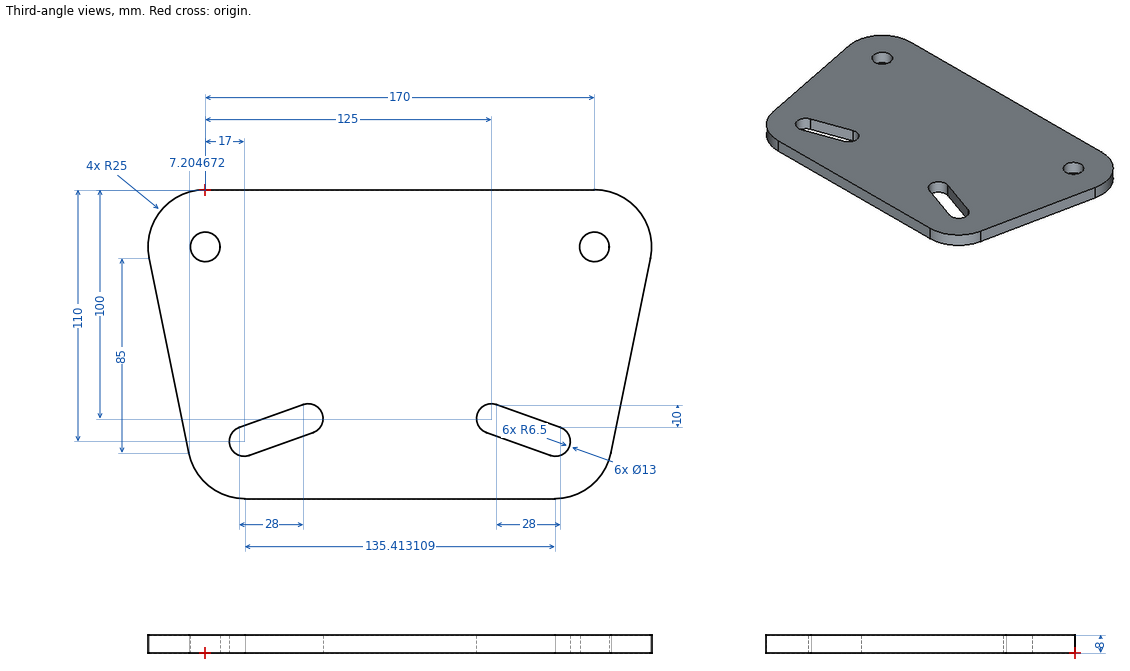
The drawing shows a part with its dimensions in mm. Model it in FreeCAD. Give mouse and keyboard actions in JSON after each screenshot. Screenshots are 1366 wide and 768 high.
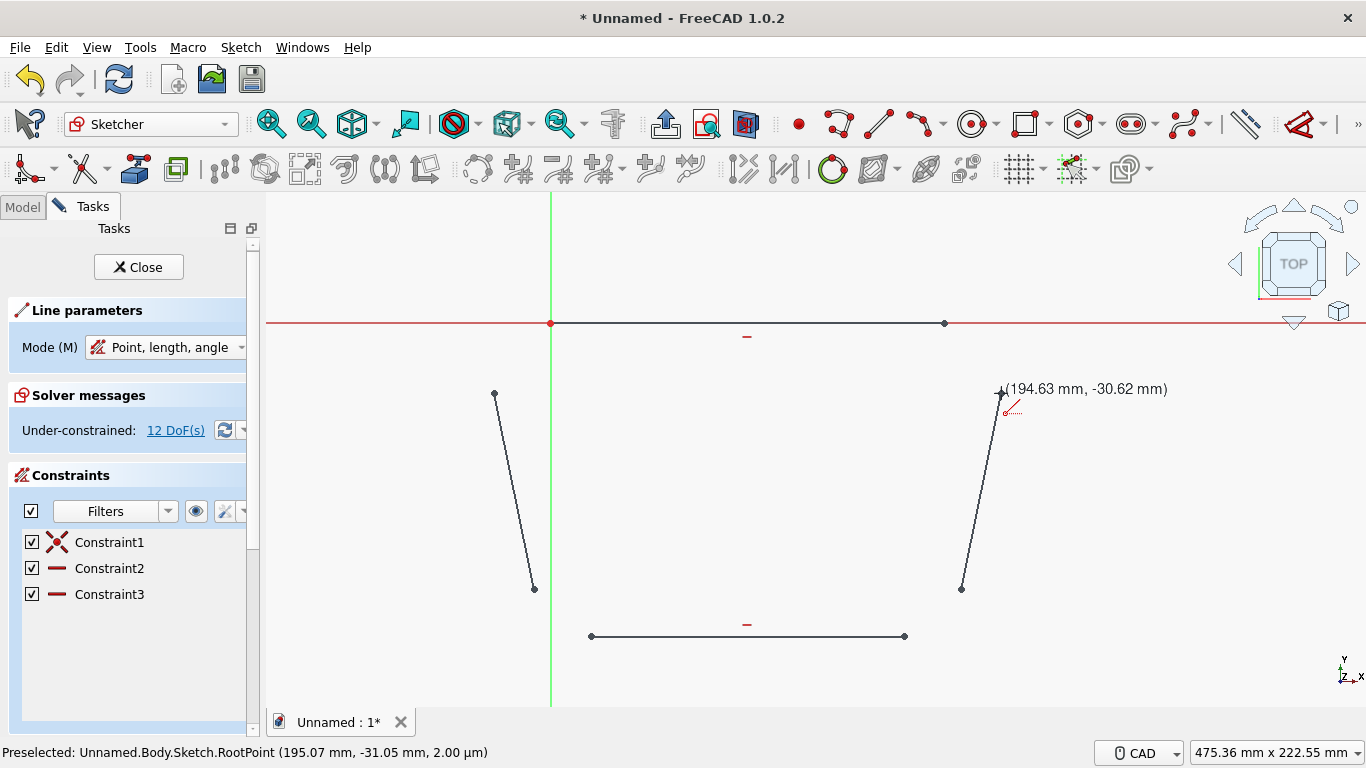
{"action": "left_click", "coordinate": [920, 124]}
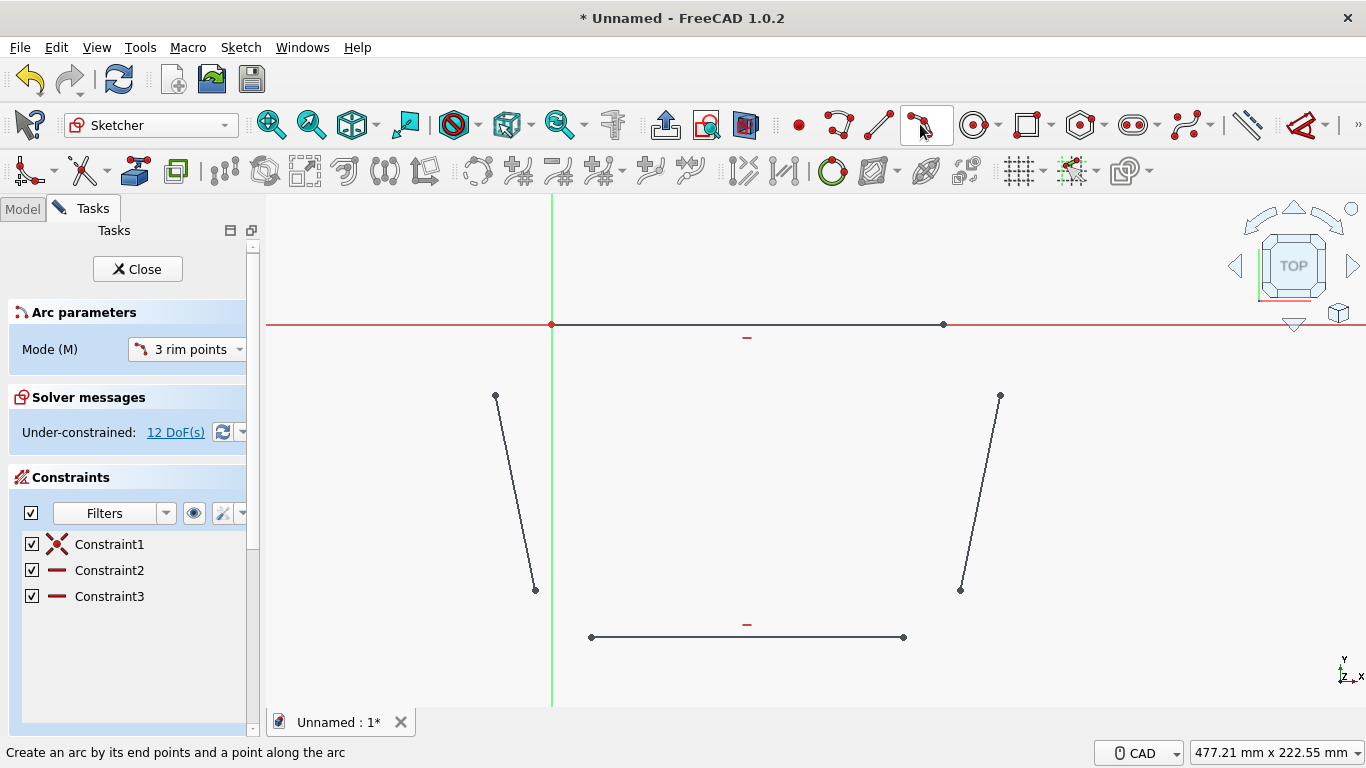
{"action": "left_click", "coordinate": [552, 325]}
{"action": "left_click", "coordinate": [495, 395]}
{"action": "left_click", "coordinate": [507, 346]}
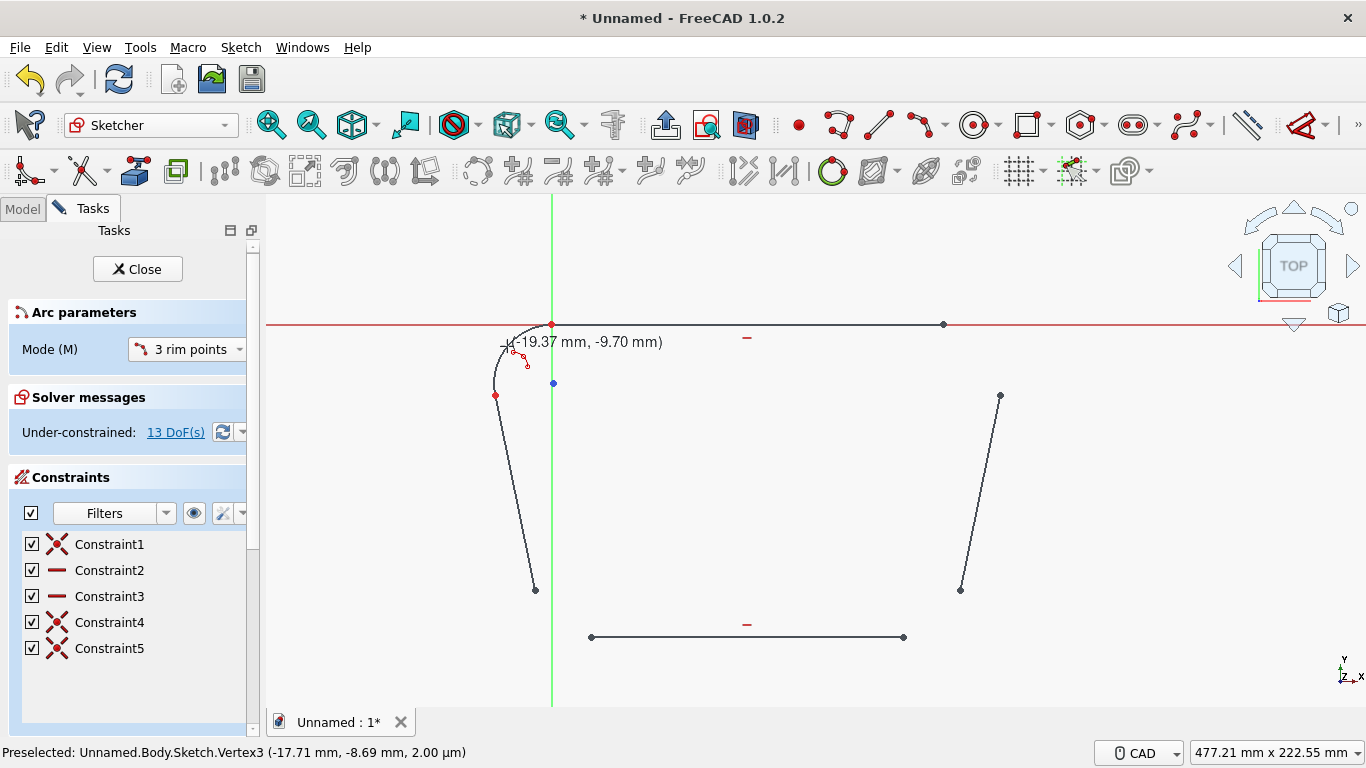
{"action": "left_click", "coordinate": [535, 590]}
{"action": "left_click", "coordinate": [592, 637]}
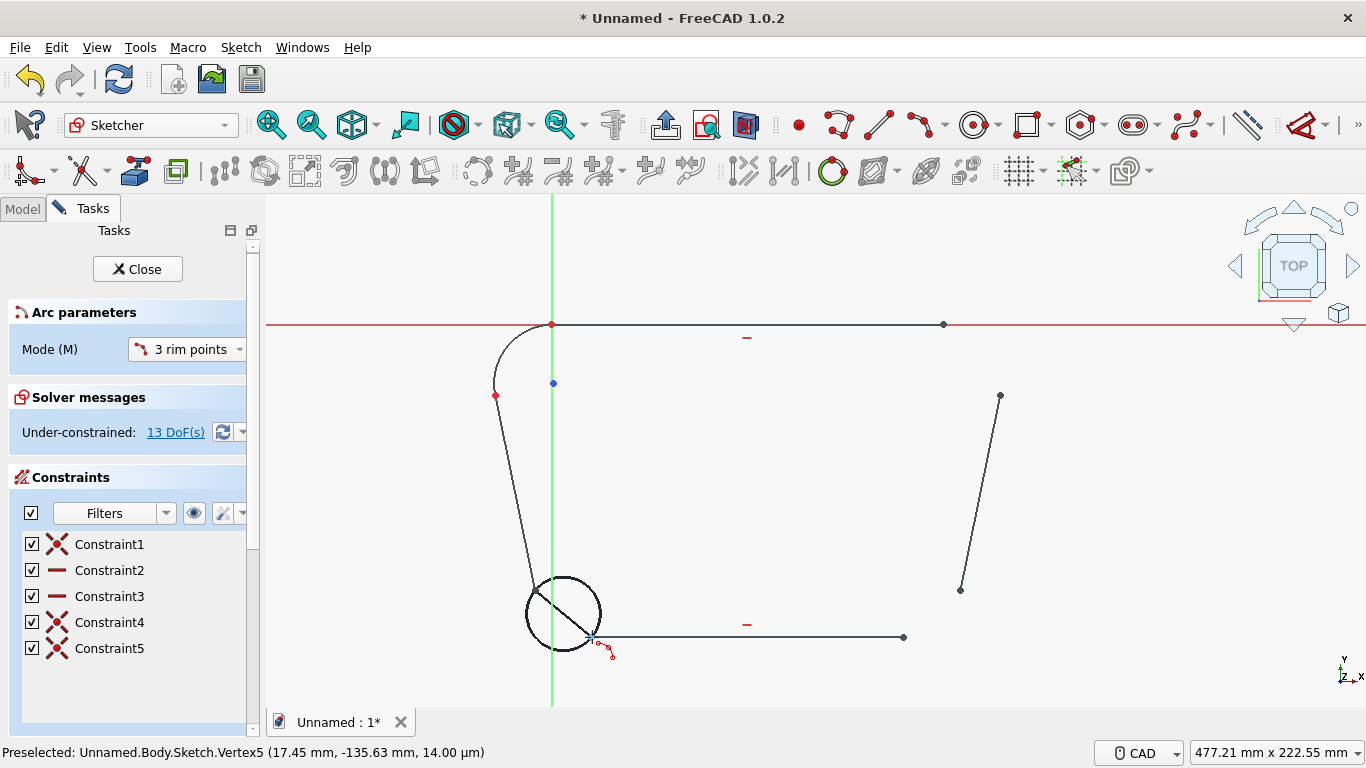
{"action": "scroll", "coordinate": [568, 631], "scroll_direction": "up", "scroll_amount": 2}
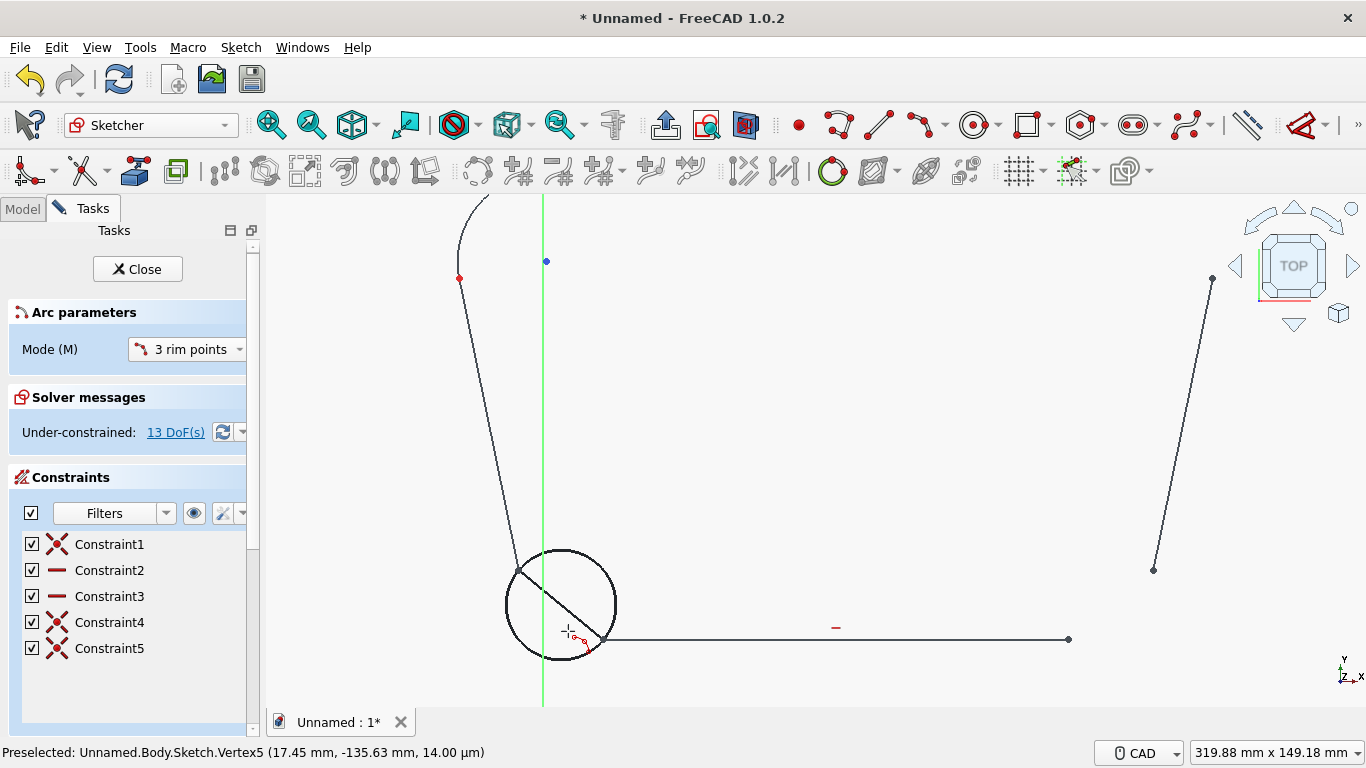
{"action": "left_click", "coordinate": [569, 631]}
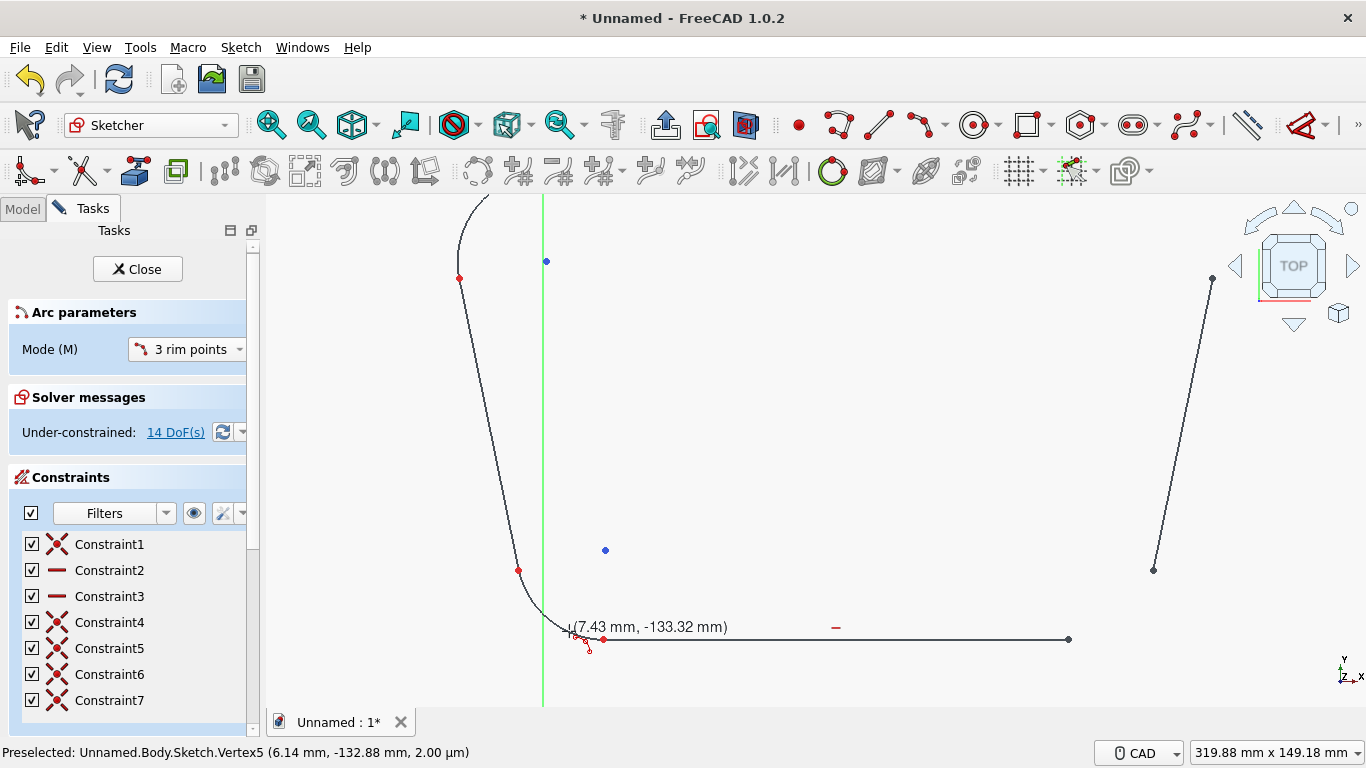
{"action": "left_click", "coordinate": [1069, 640]}
{"action": "left_click", "coordinate": [1153, 570]}
{"action": "left_click", "coordinate": [1123, 618]}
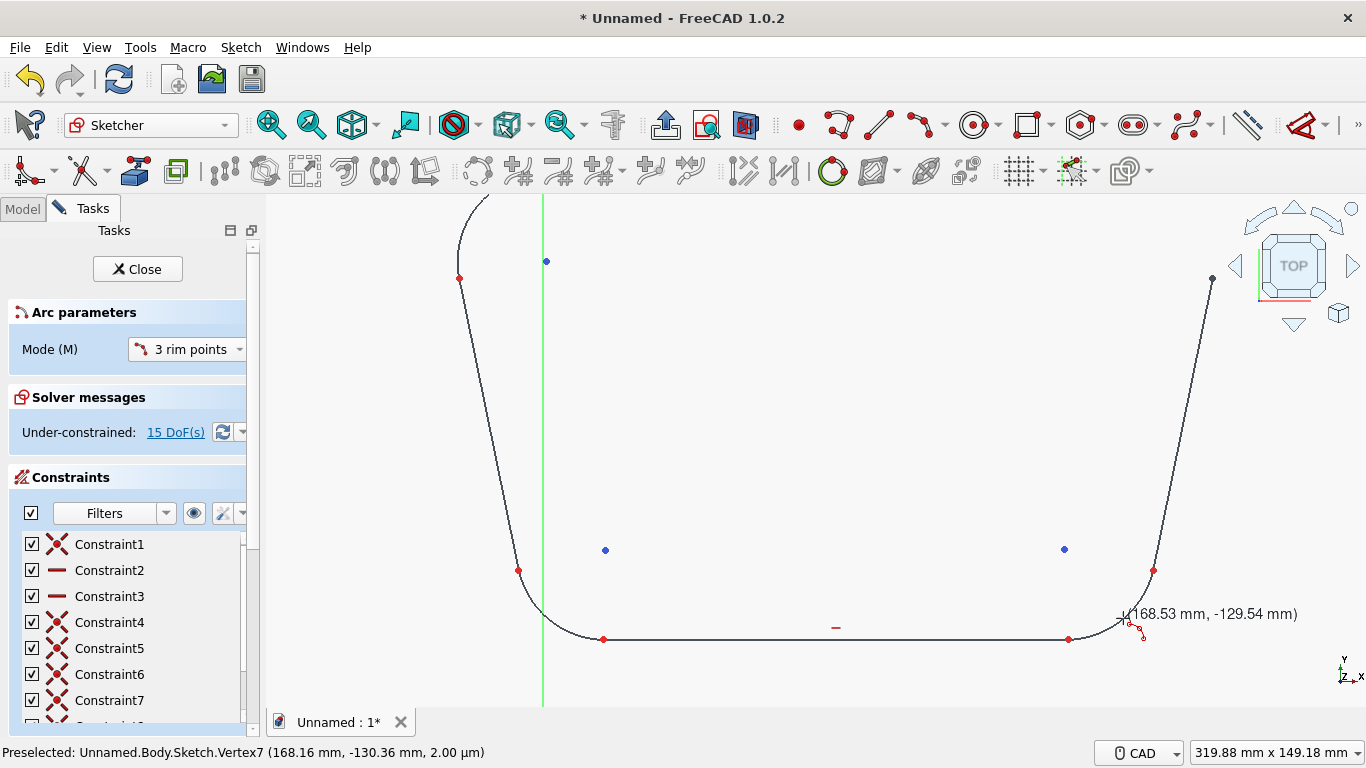
{"action": "scroll", "coordinate": [568, 542], "scroll_direction": "down", "scroll_amount": 2}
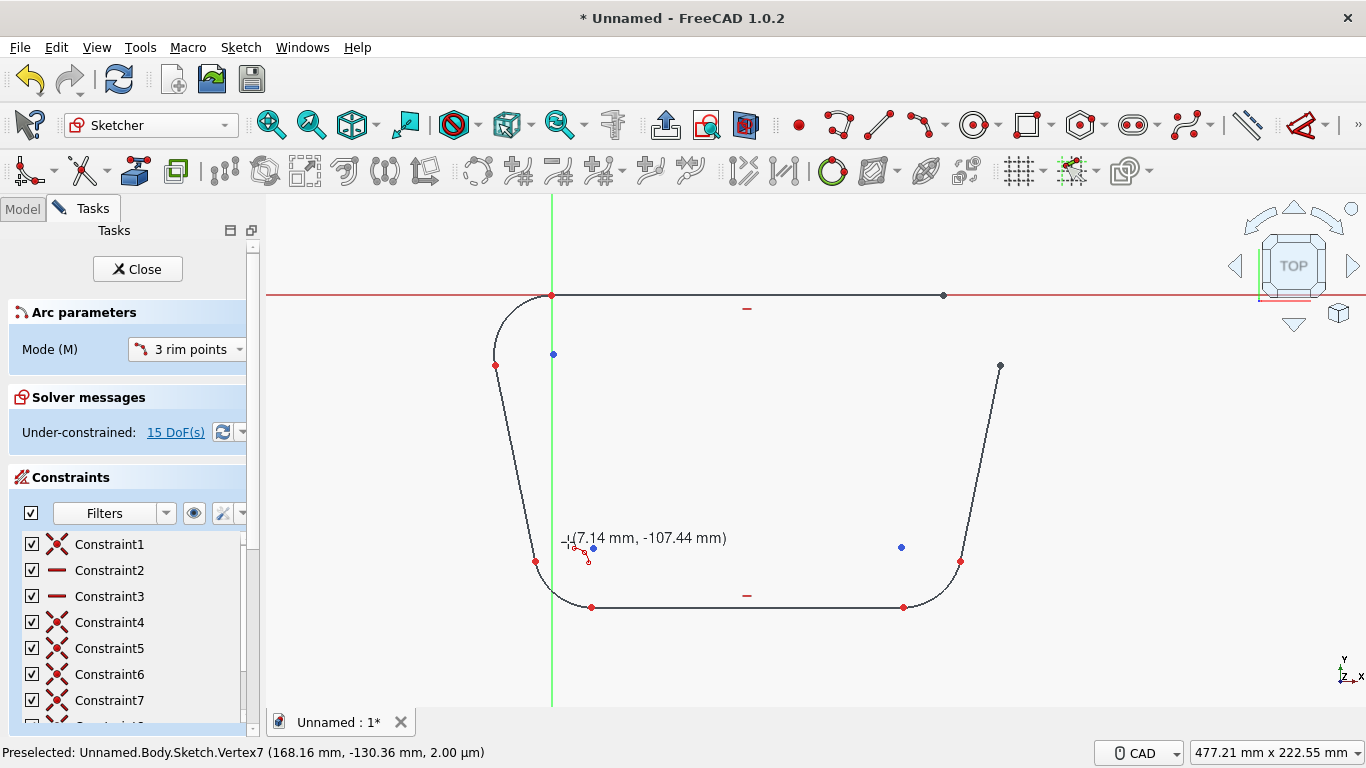
{"action": "left_click", "coordinate": [1000, 366]}
{"action": "left_click", "coordinate": [944, 295]}
{"action": "left_click", "coordinate": [988, 316]}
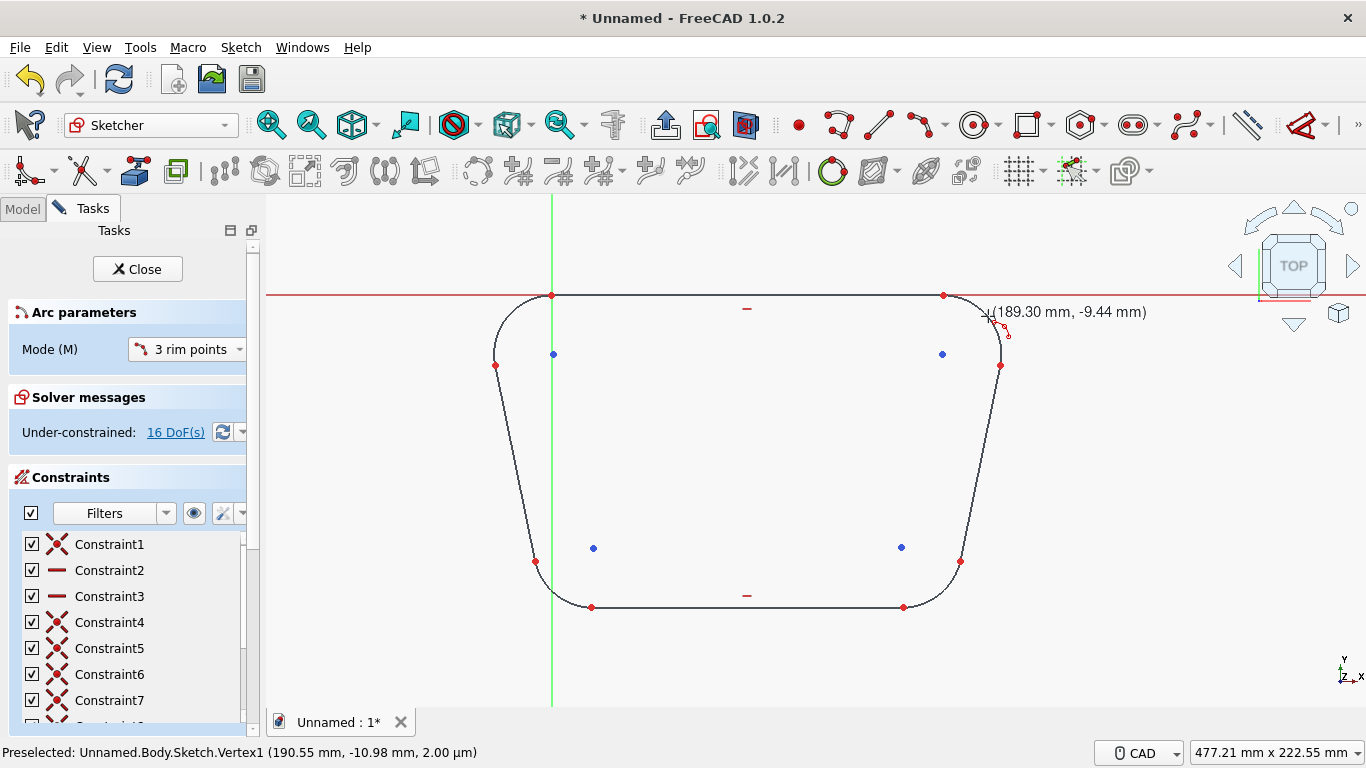
{"action": "left_click", "coordinate": [1134, 126]}